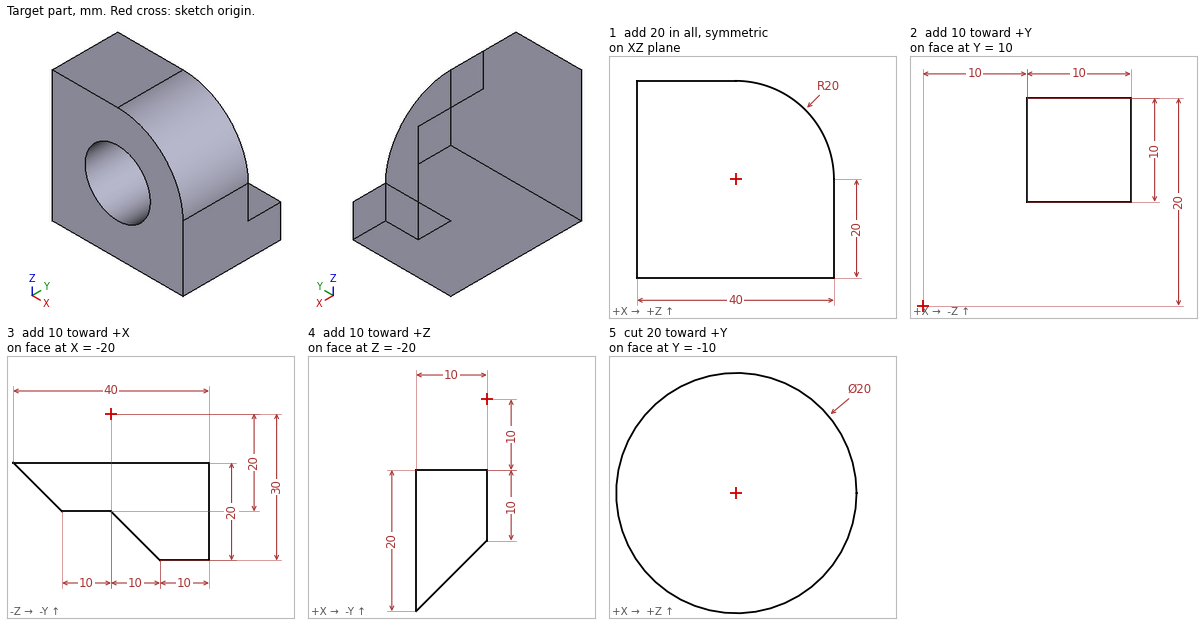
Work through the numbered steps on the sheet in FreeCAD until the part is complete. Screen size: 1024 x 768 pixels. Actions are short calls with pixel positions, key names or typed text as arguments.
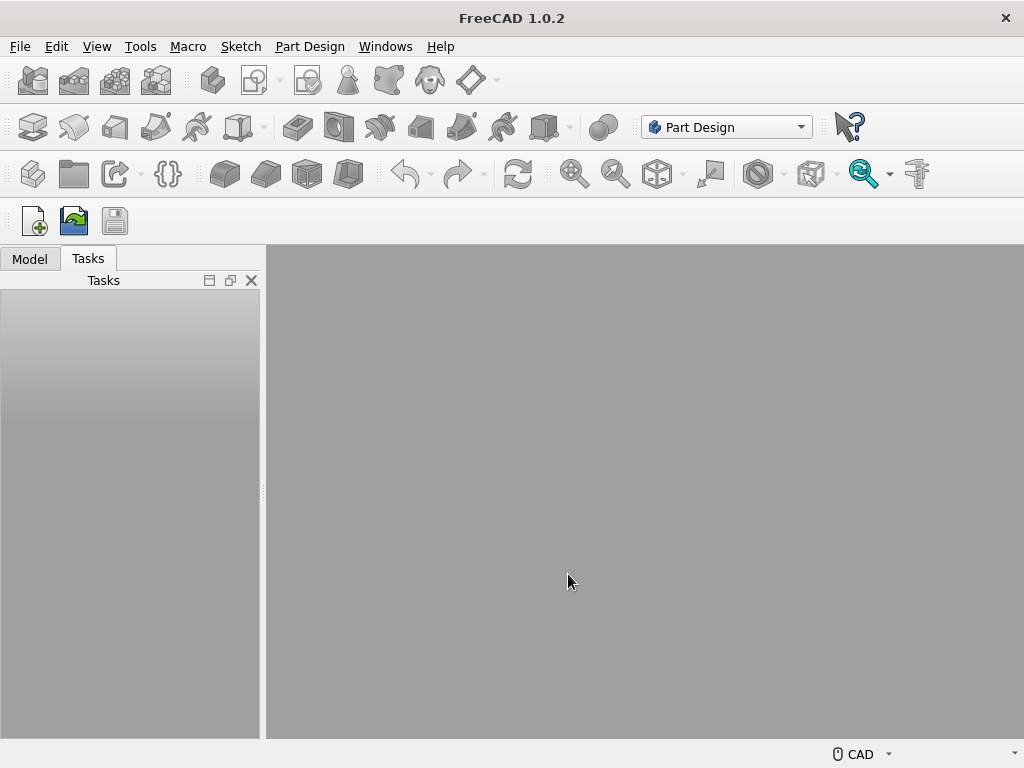
click(33, 222)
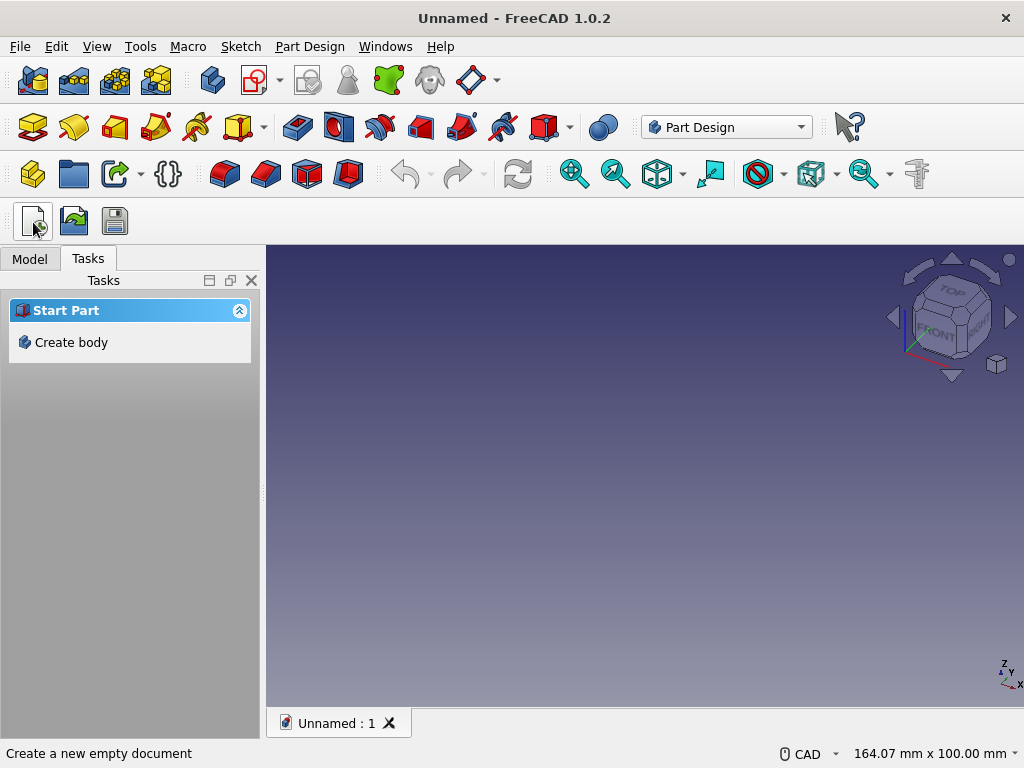
click(254, 80)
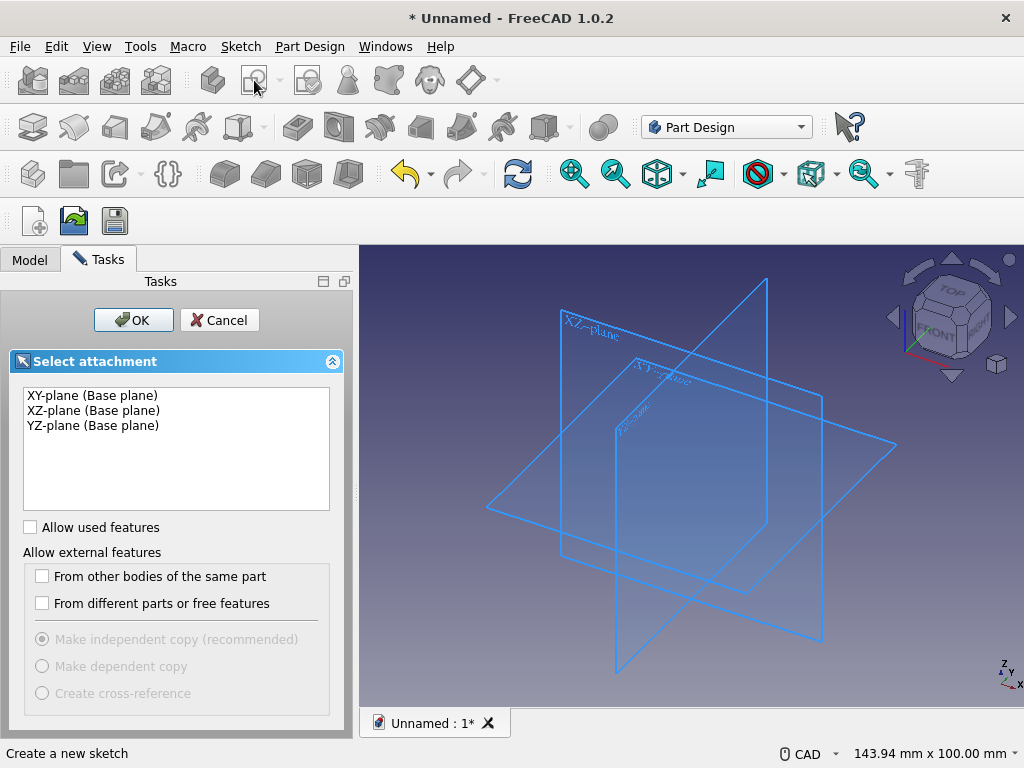
click(84, 410)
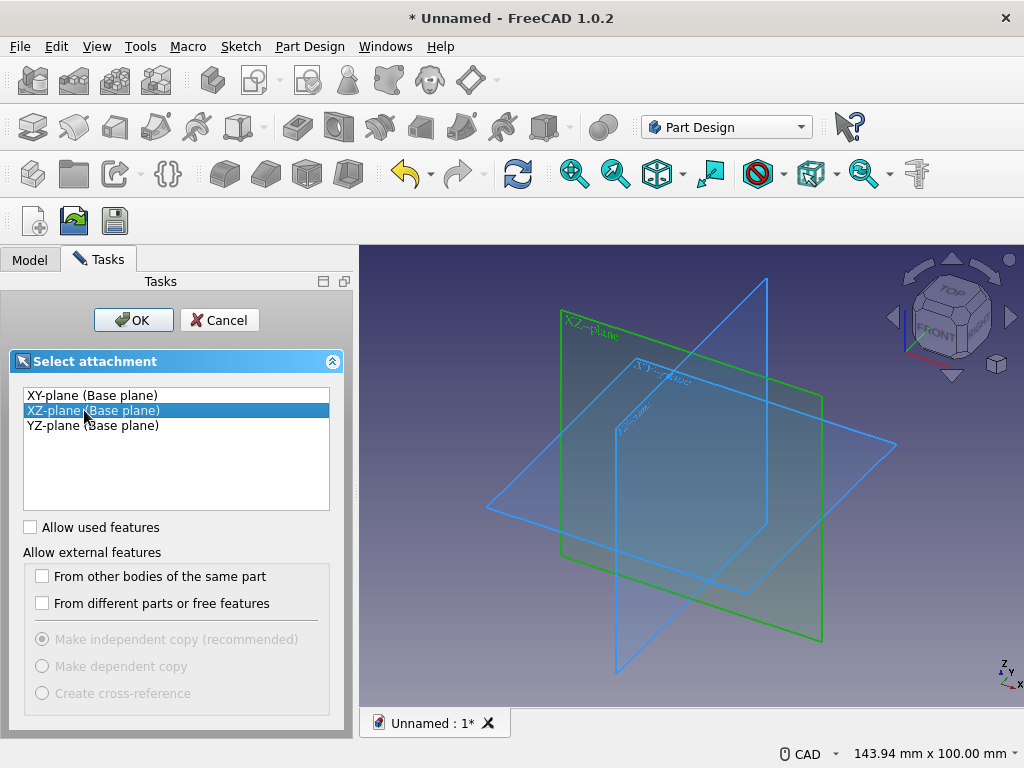
click(134, 320)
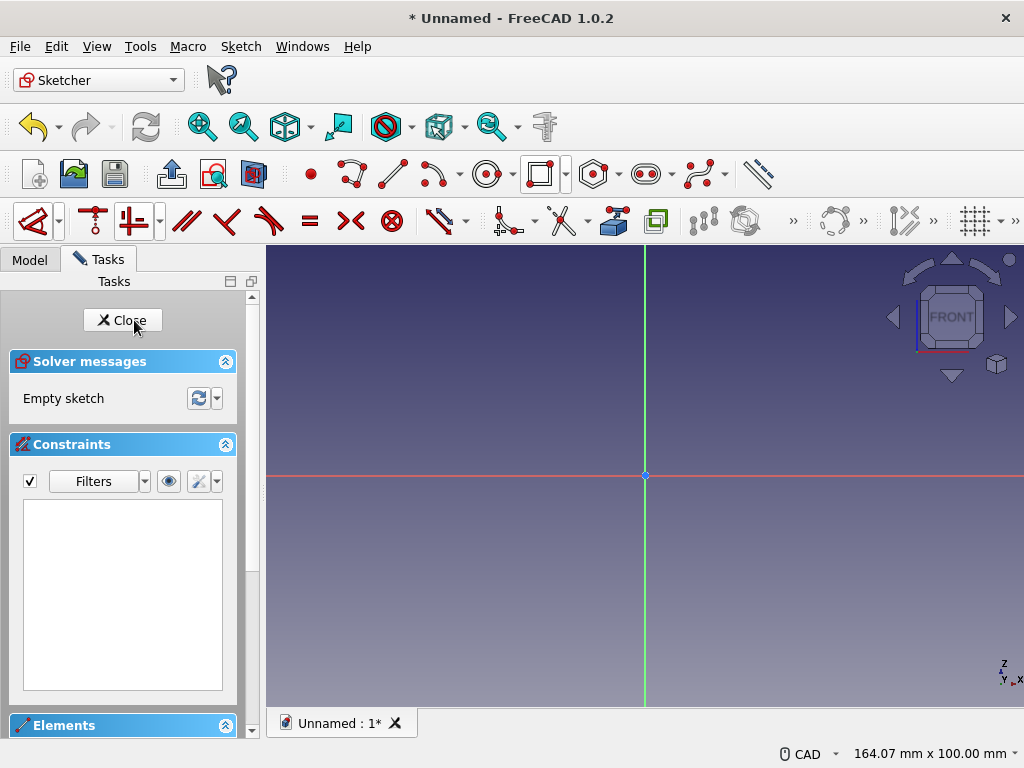
scroll(784, 476, up, 2)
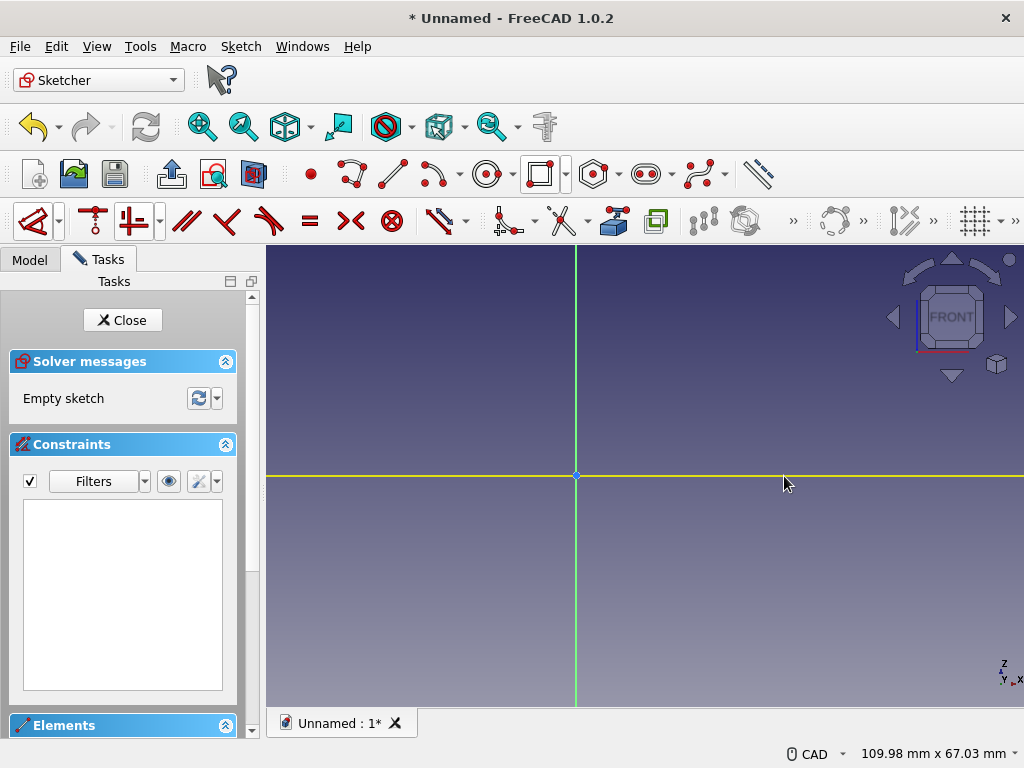
click(352, 174)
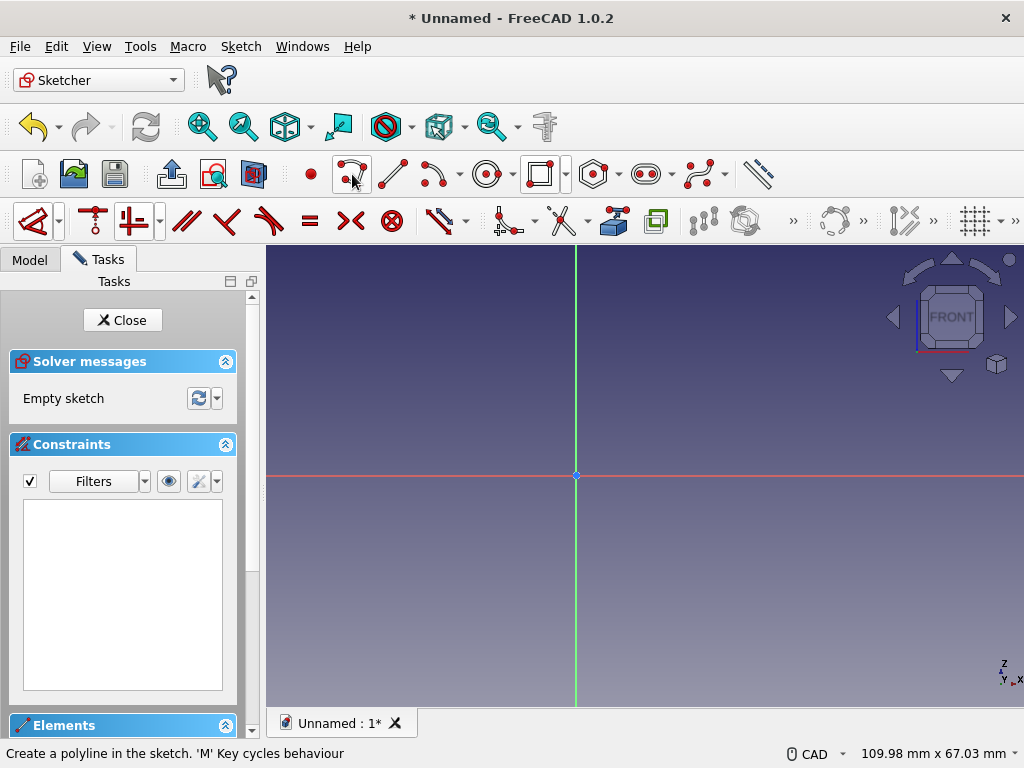
click(714, 476)
click(714, 614)
click(438, 614)
click(438, 338)
click(576, 338)
right_click(576, 338)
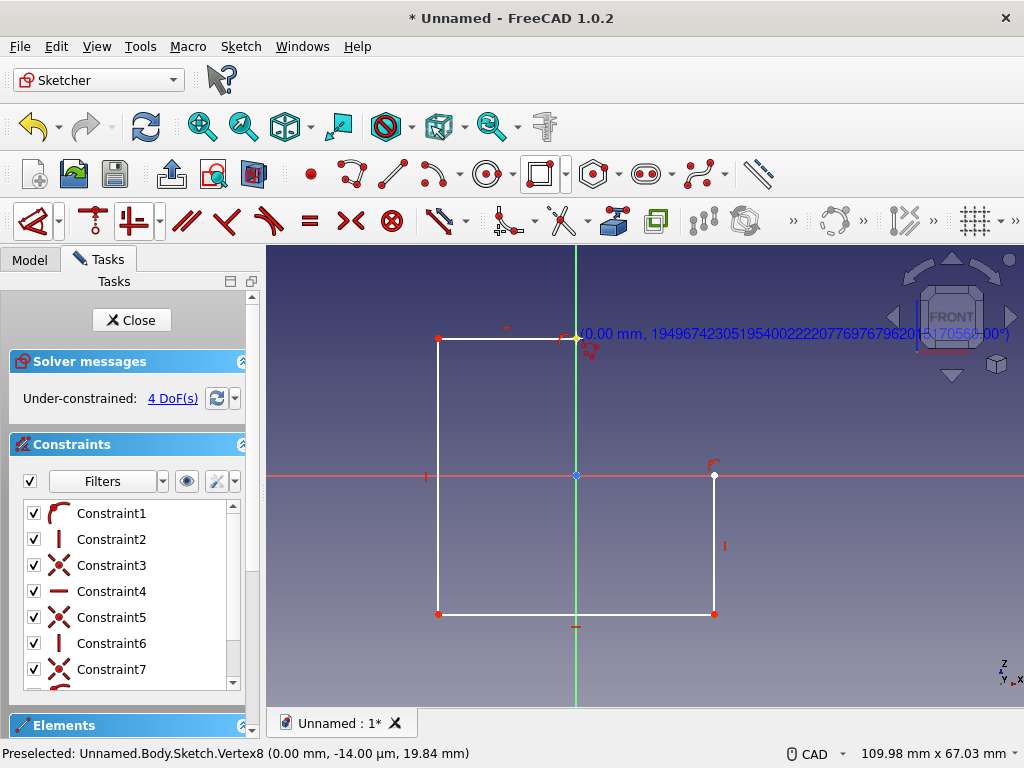
key(g)
key(3)
key(a)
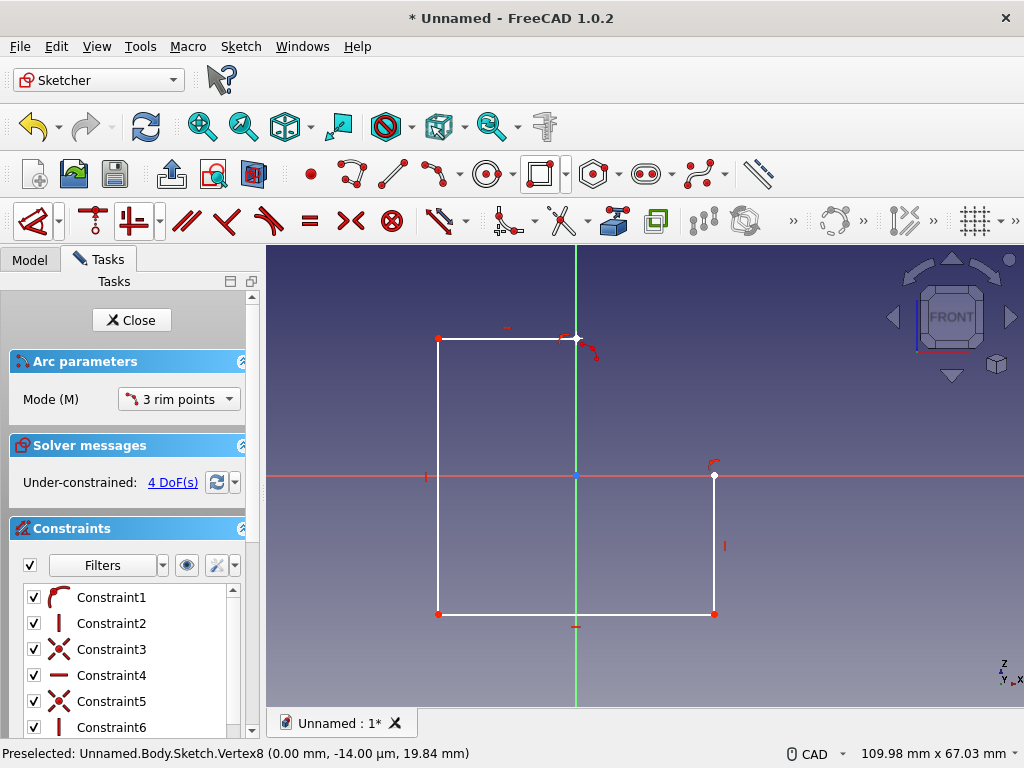
click(576, 339)
click(714, 476)
click(674, 378)
key(Escape)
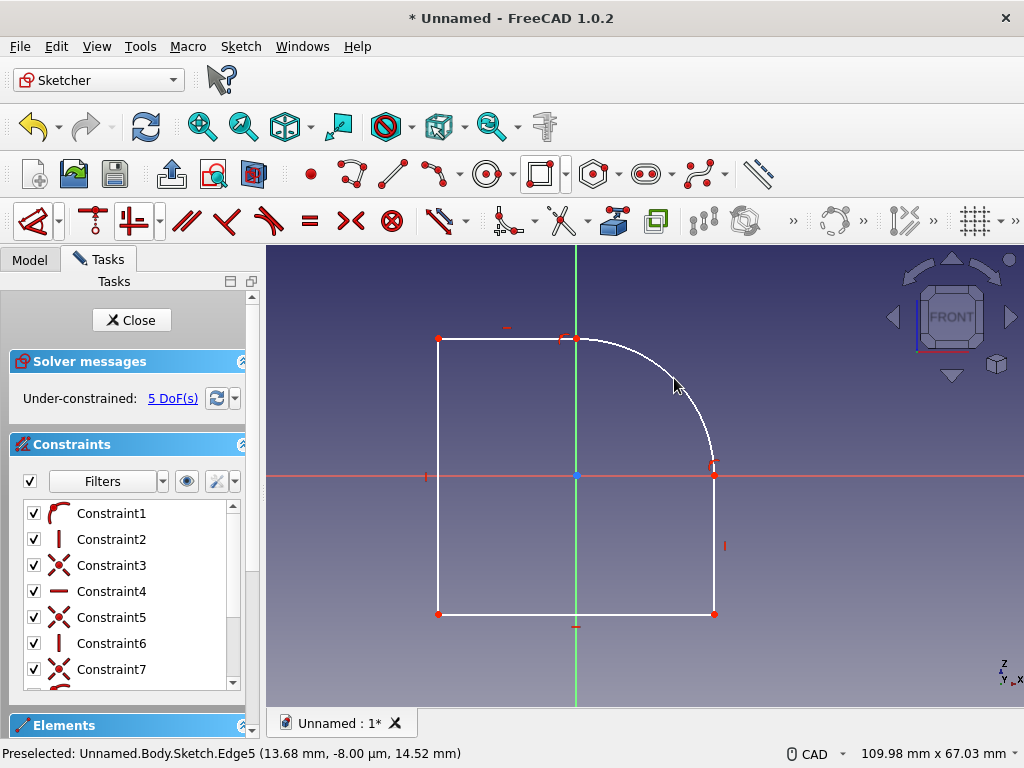
click(714, 518)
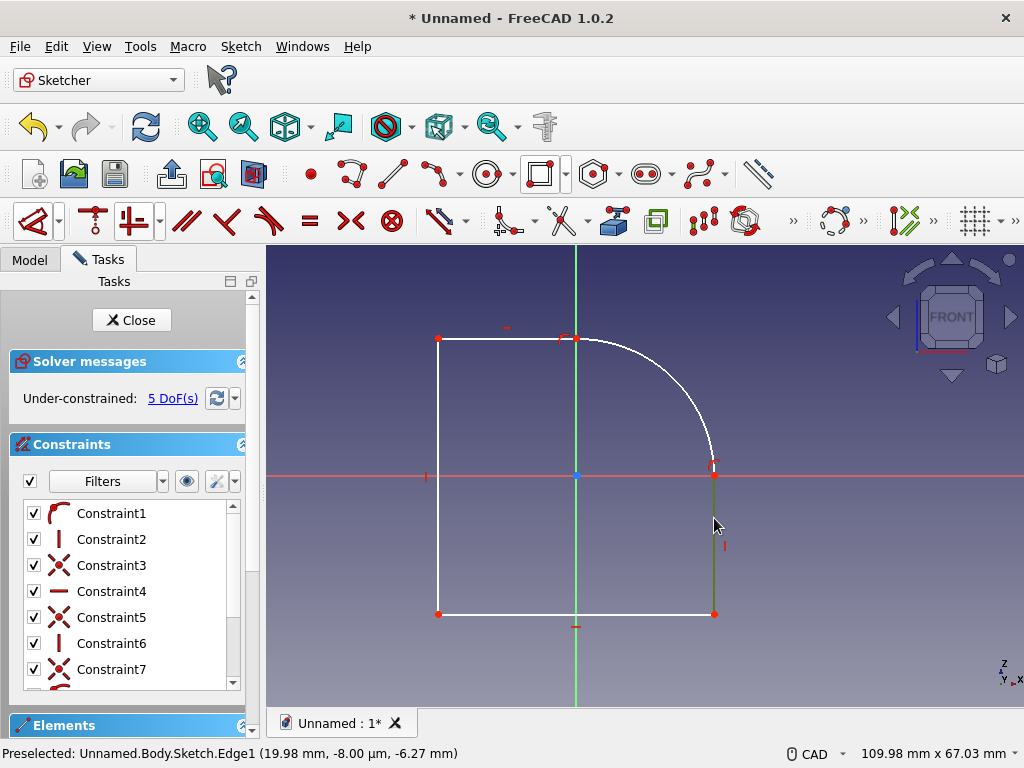
click(699, 413)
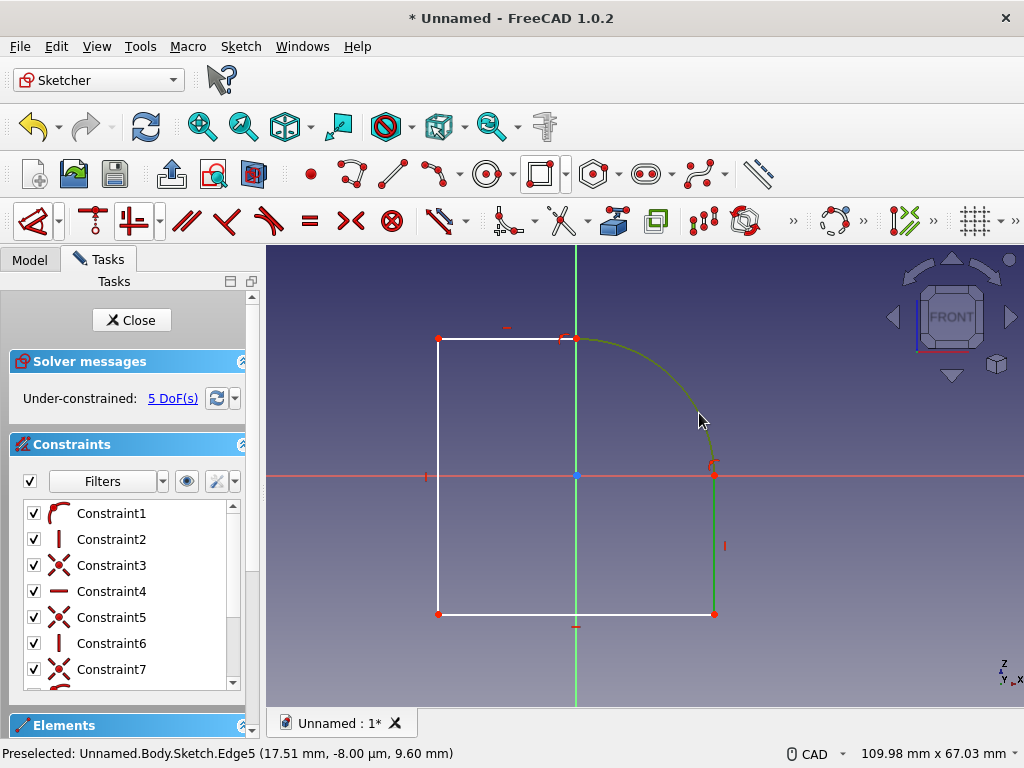
click(269, 222)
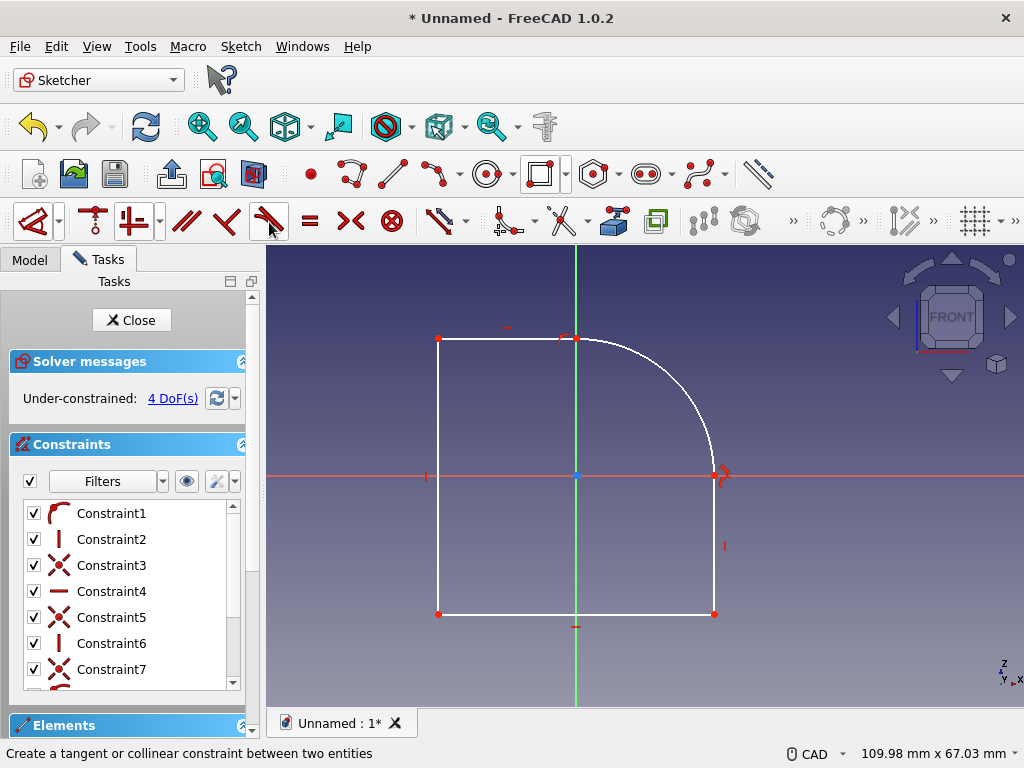
click(479, 339)